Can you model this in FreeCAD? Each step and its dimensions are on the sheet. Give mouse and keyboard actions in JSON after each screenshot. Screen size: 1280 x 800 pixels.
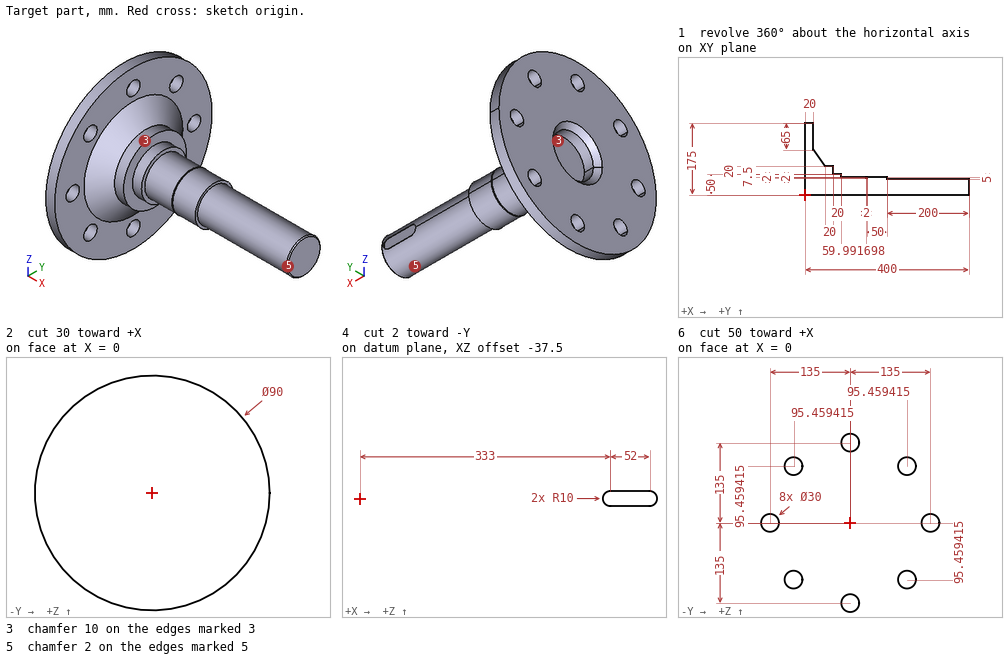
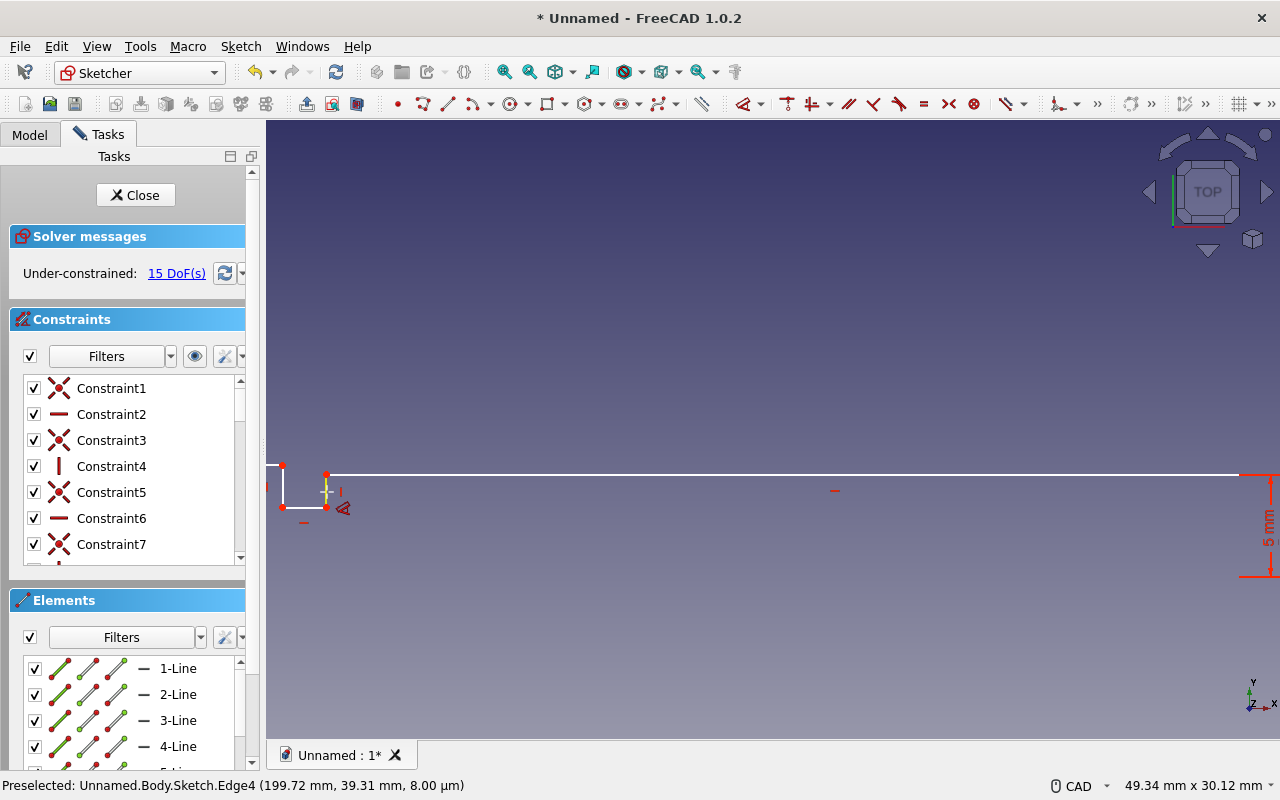
{"action": "left_click", "coordinate": [326, 491]}
{"action": "left_click", "coordinate": [360, 491]}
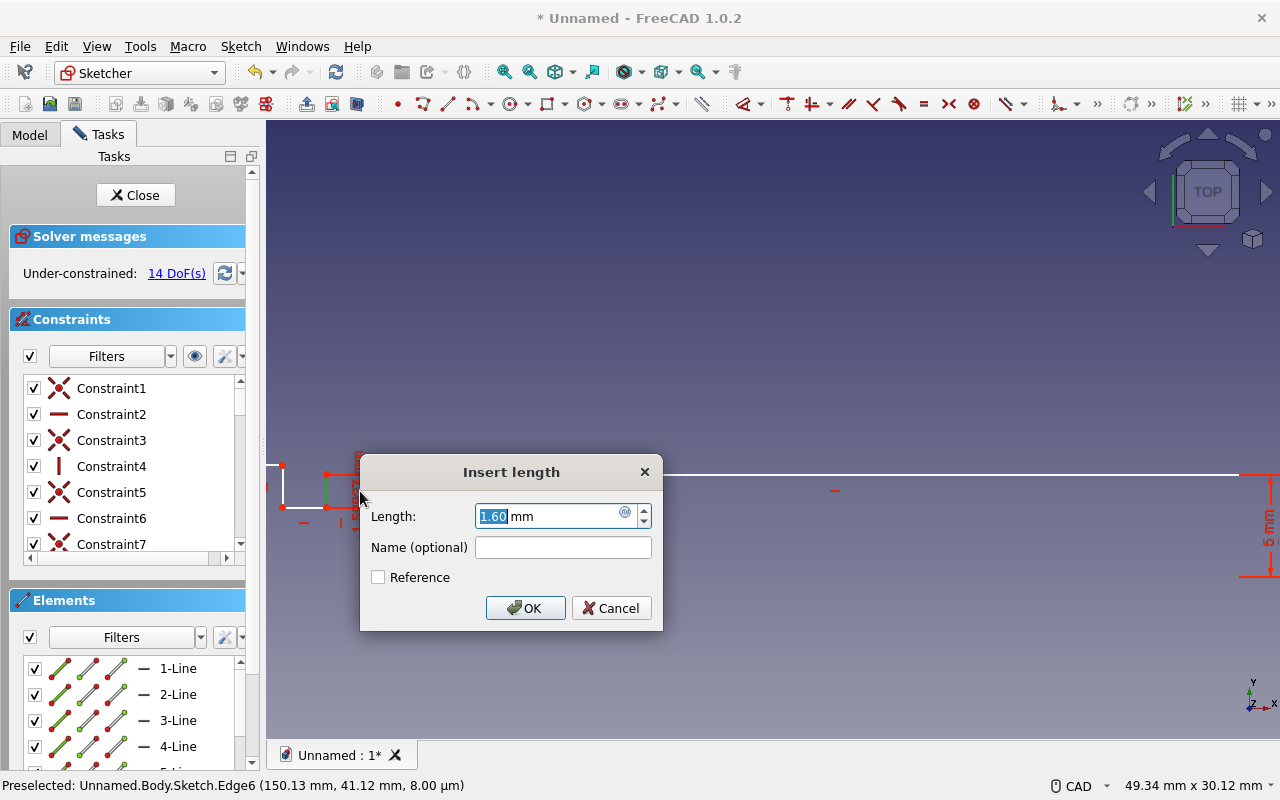
{"action": "type", "text": "2"}
{"action": "key", "text": "Return"}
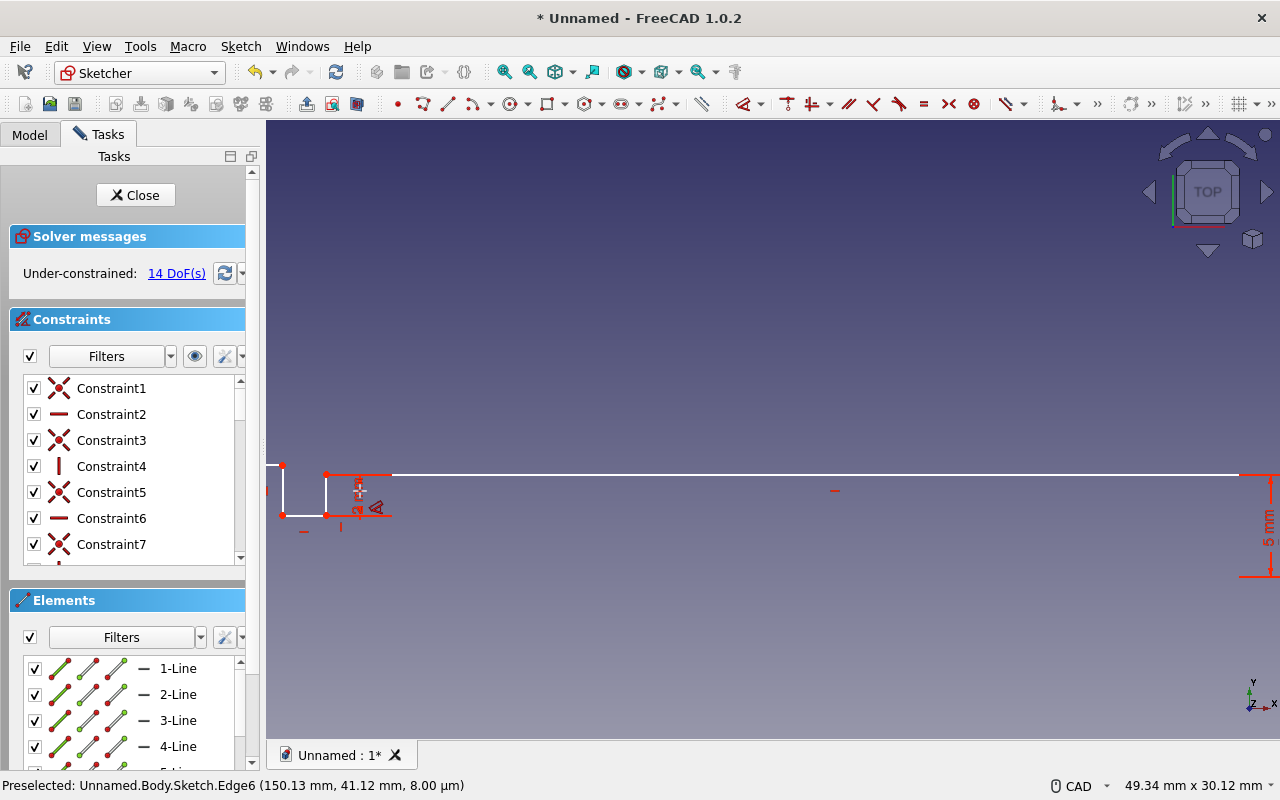
{"action": "left_click", "coordinate": [313, 516]}
{"action": "left_click", "coordinate": [310, 550]}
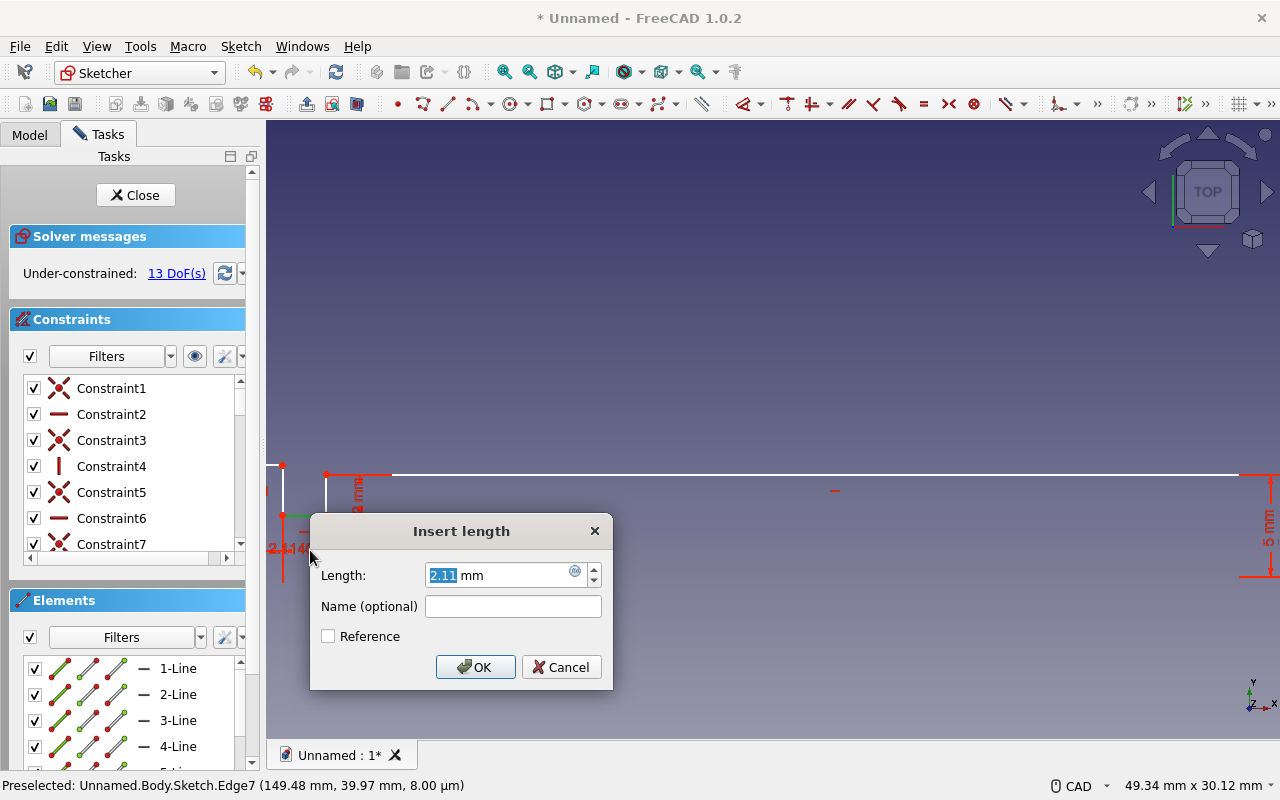
{"action": "type", "text": "2"}
{"action": "key", "text": "Return"}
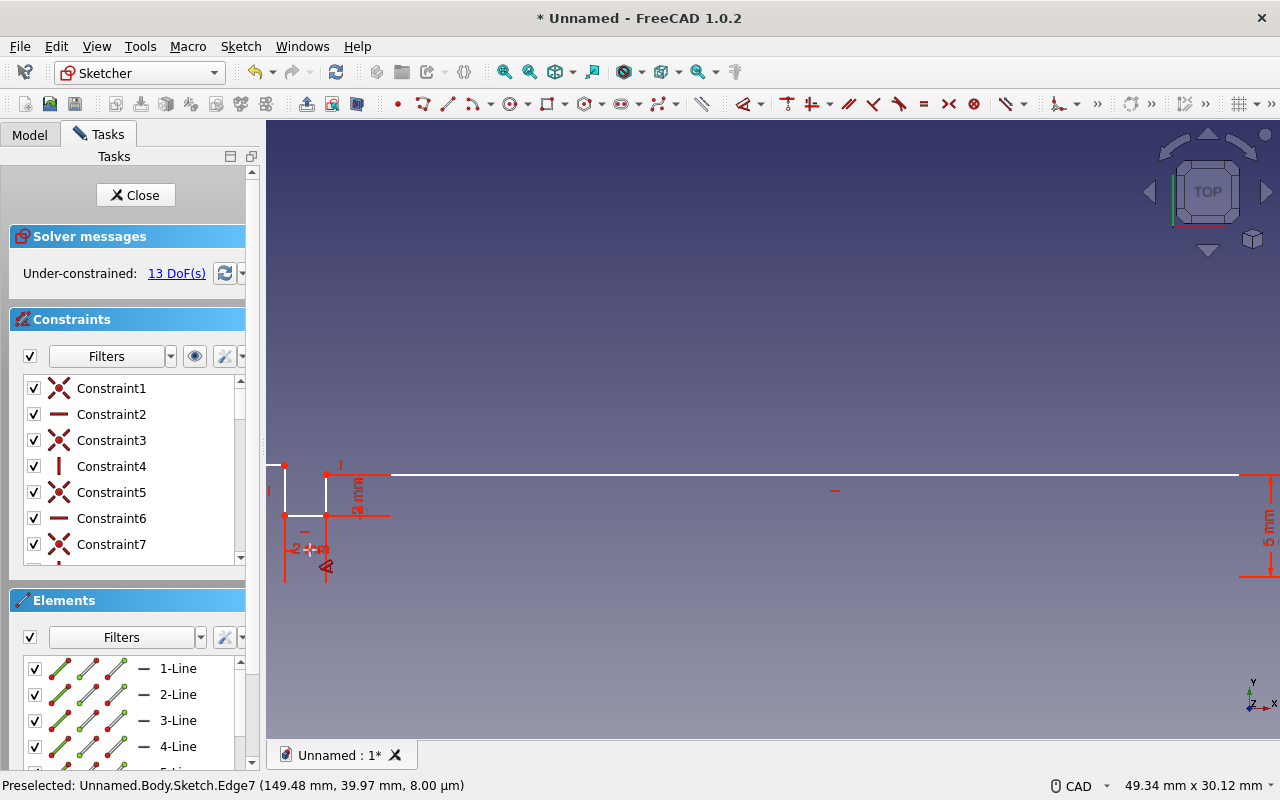
{"action": "scroll", "coordinate": [653, 501], "scroll_direction": "down", "scroll_amount": 13}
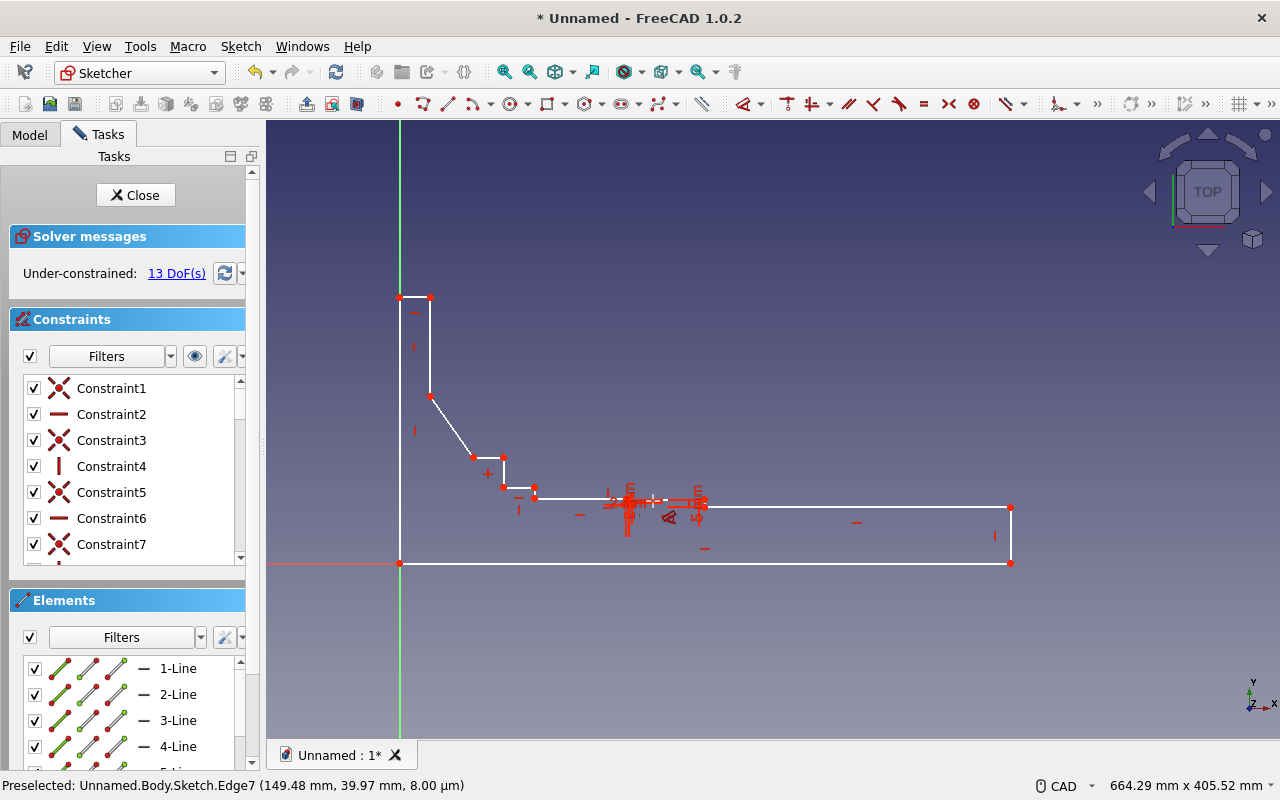
{"action": "scroll", "coordinate": [626, 502], "scroll_direction": "up", "scroll_amount": 13}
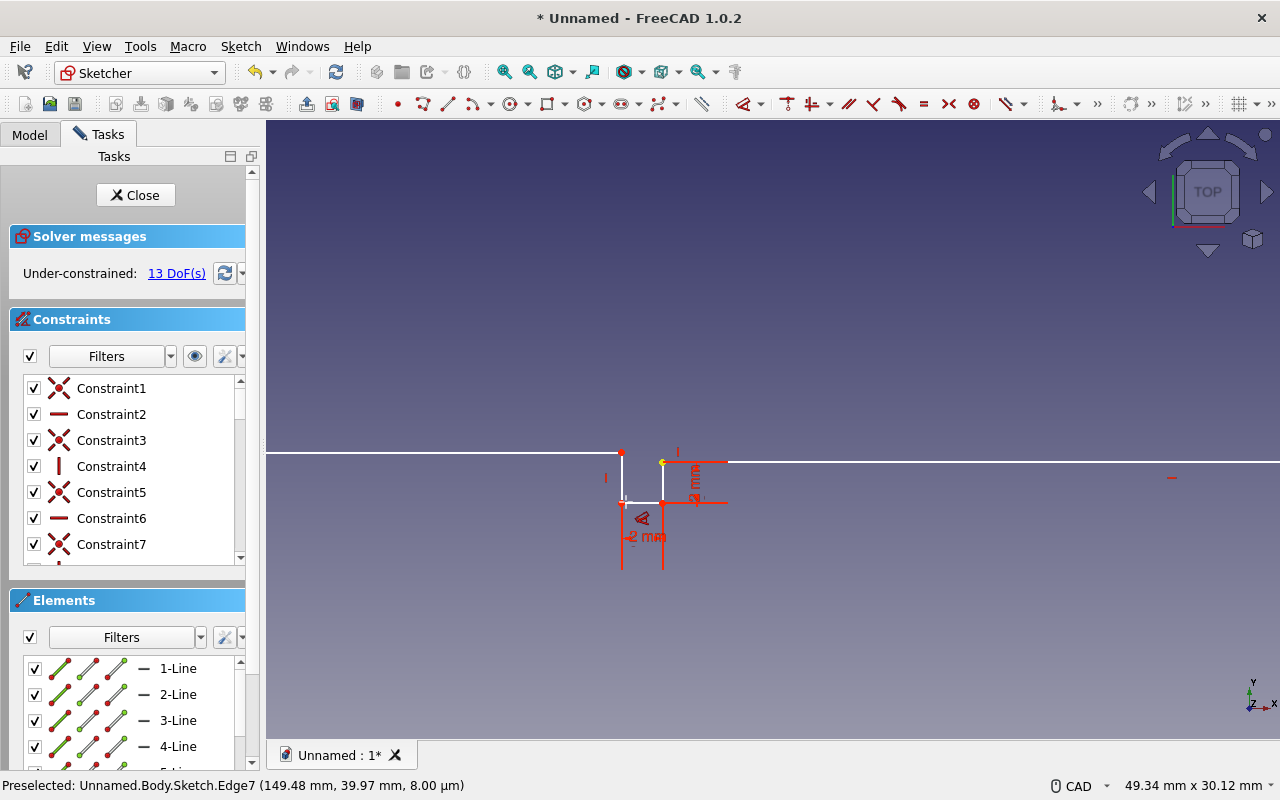
{"action": "left_click", "coordinate": [622, 488]}
{"action": "left_click", "coordinate": [588, 478]}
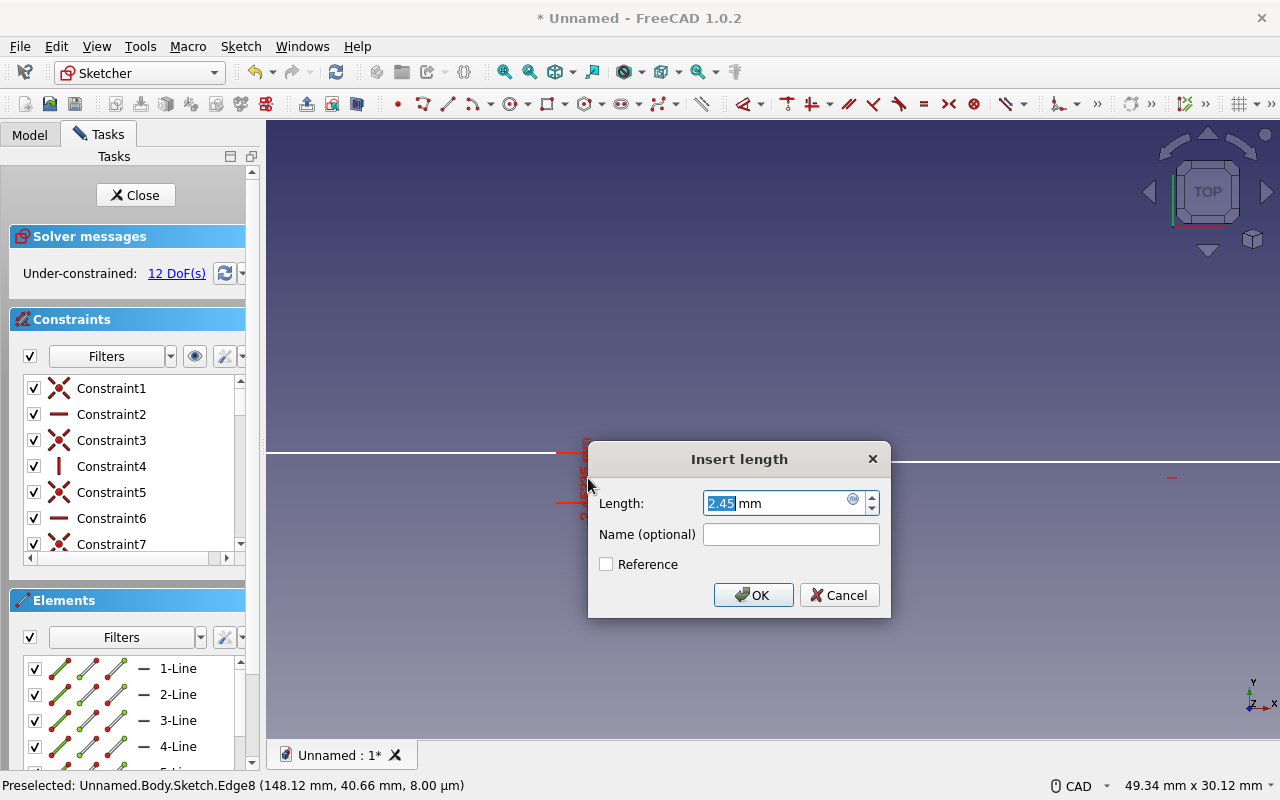
{"action": "type", "text": "2"}
{"action": "key", "text": "Return"}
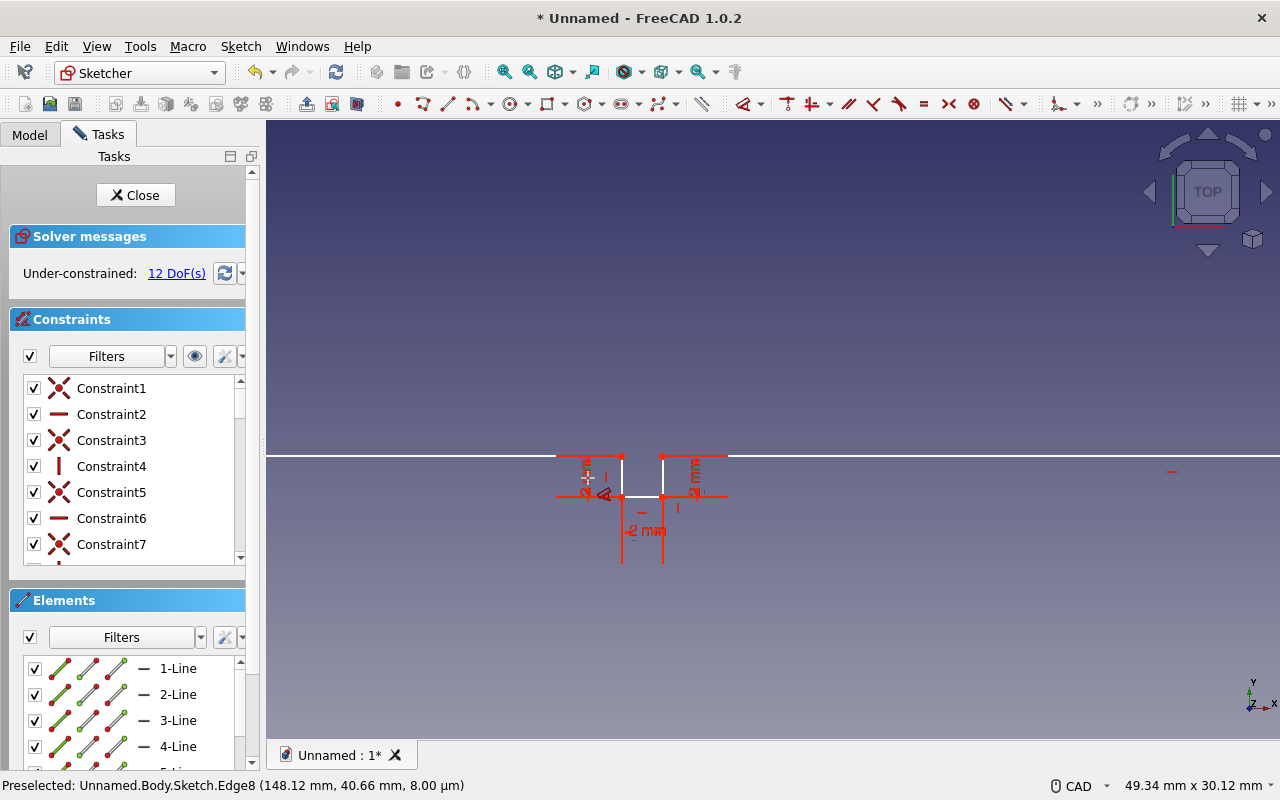
{"action": "scroll", "coordinate": [626, 502], "scroll_direction": "down", "scroll_amount": 13}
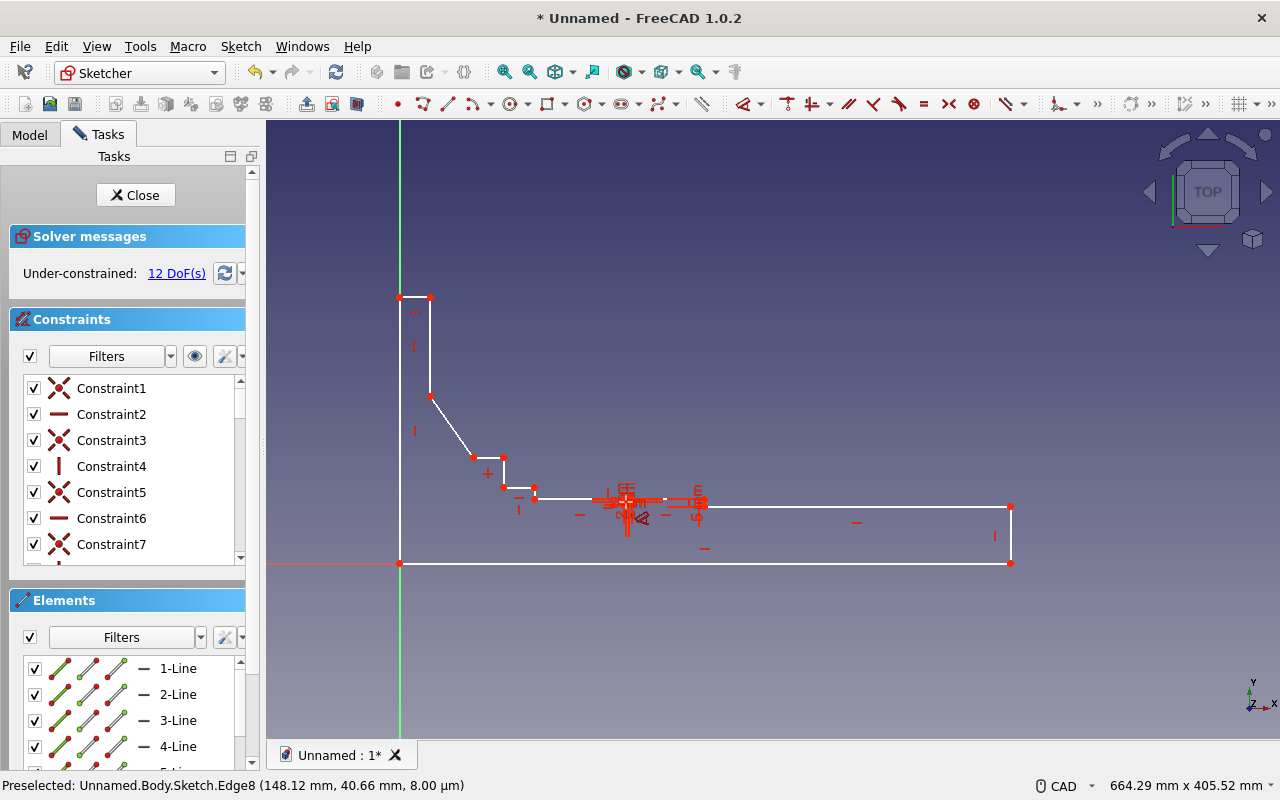
{"action": "left_click", "coordinate": [652, 499]}
{"action": "left_click", "coordinate": [667, 533]}